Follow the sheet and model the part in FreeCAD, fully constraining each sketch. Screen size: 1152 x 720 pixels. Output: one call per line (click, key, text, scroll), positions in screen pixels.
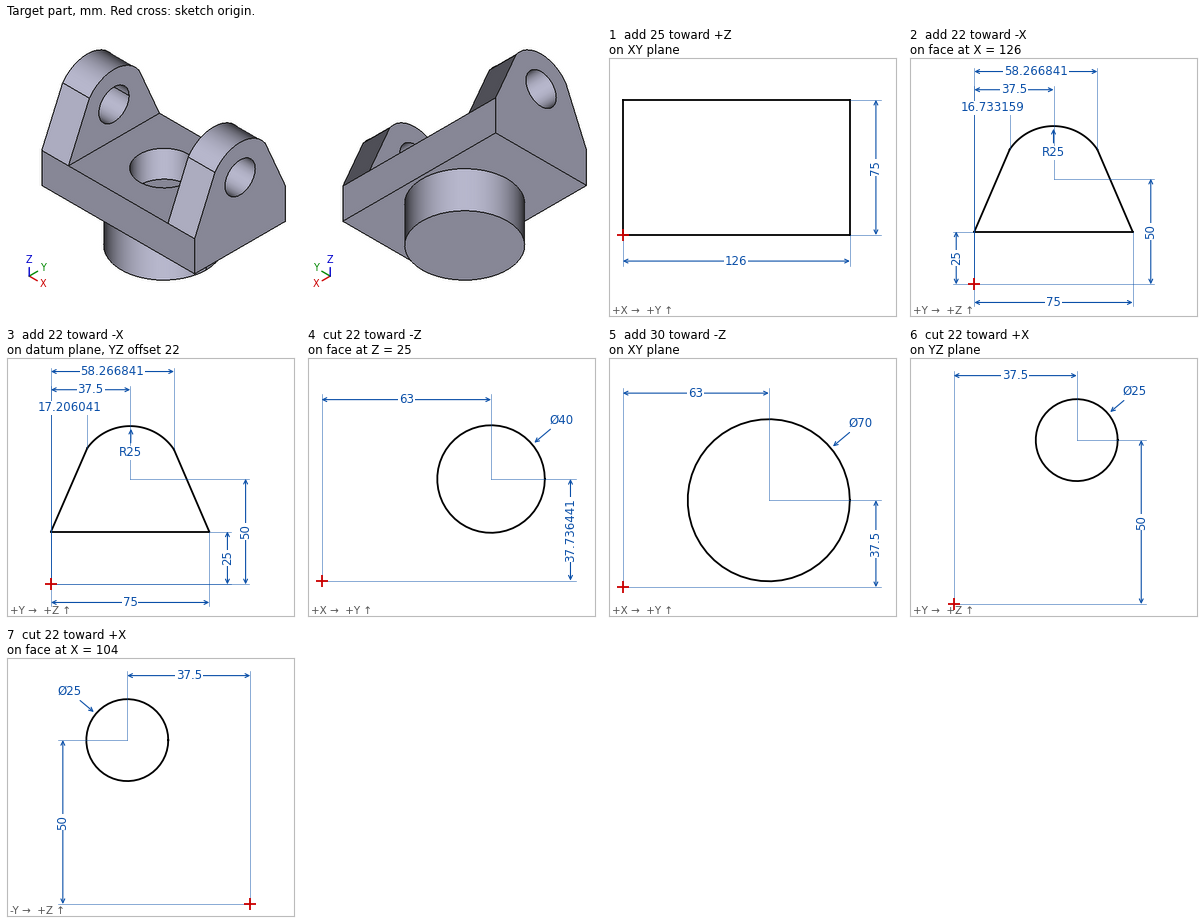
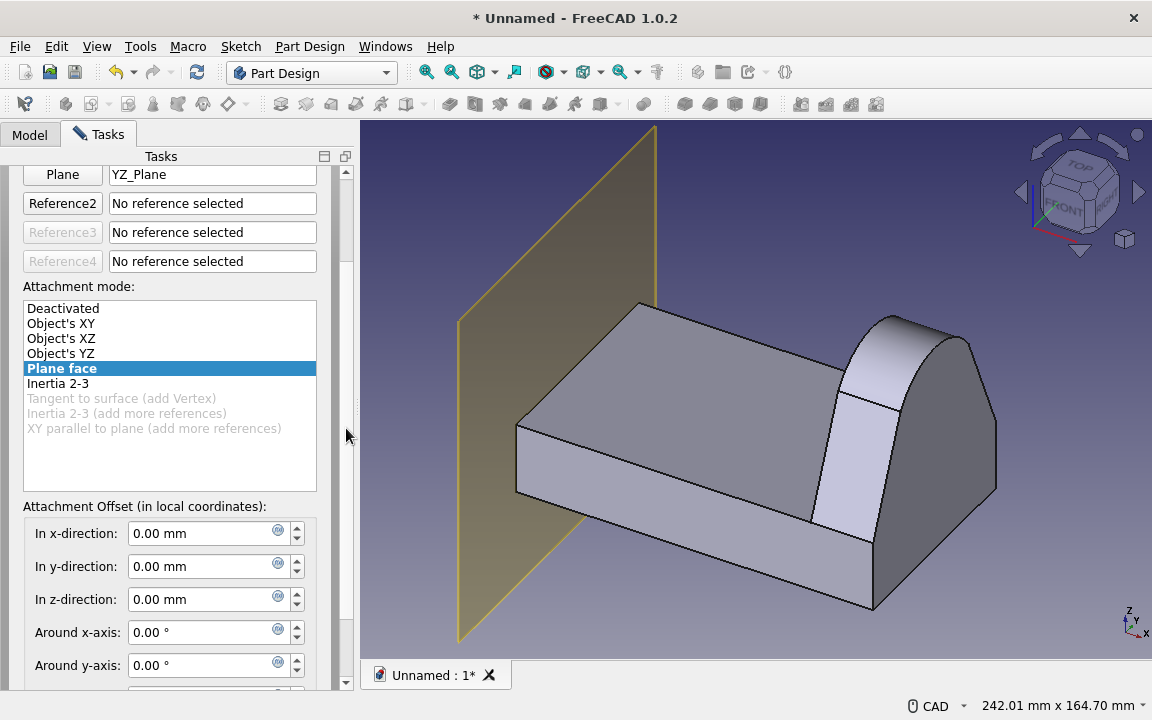
triple_click(210, 600)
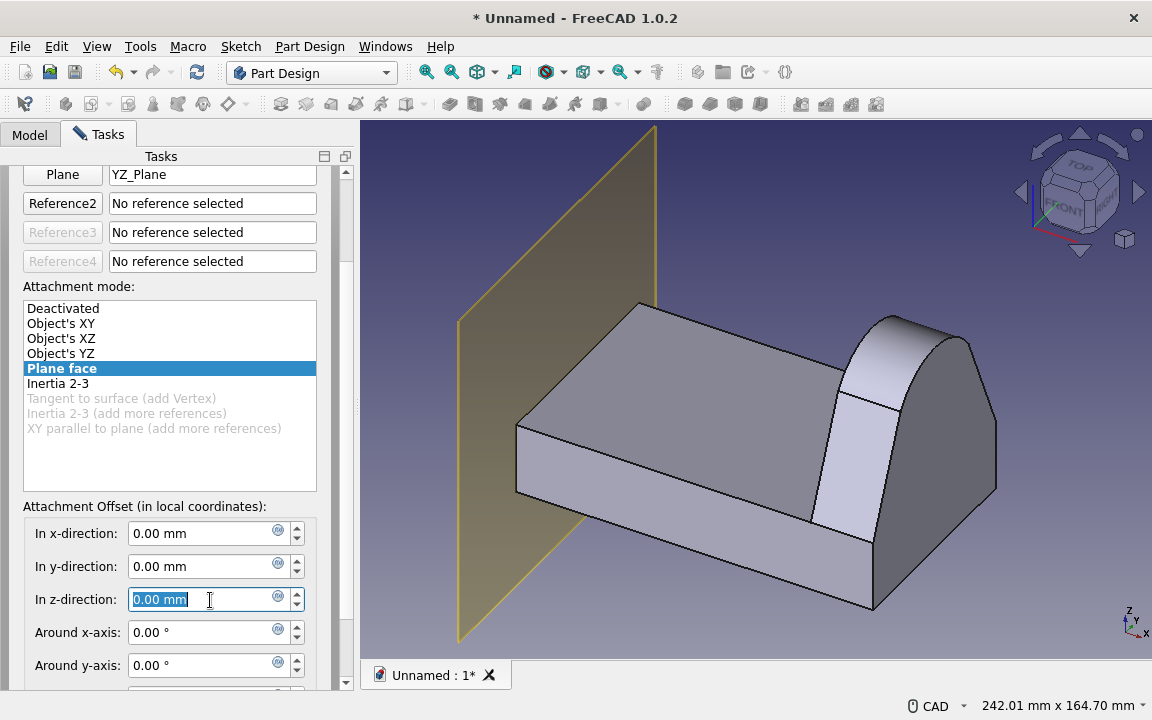
text(22)
key(Tab)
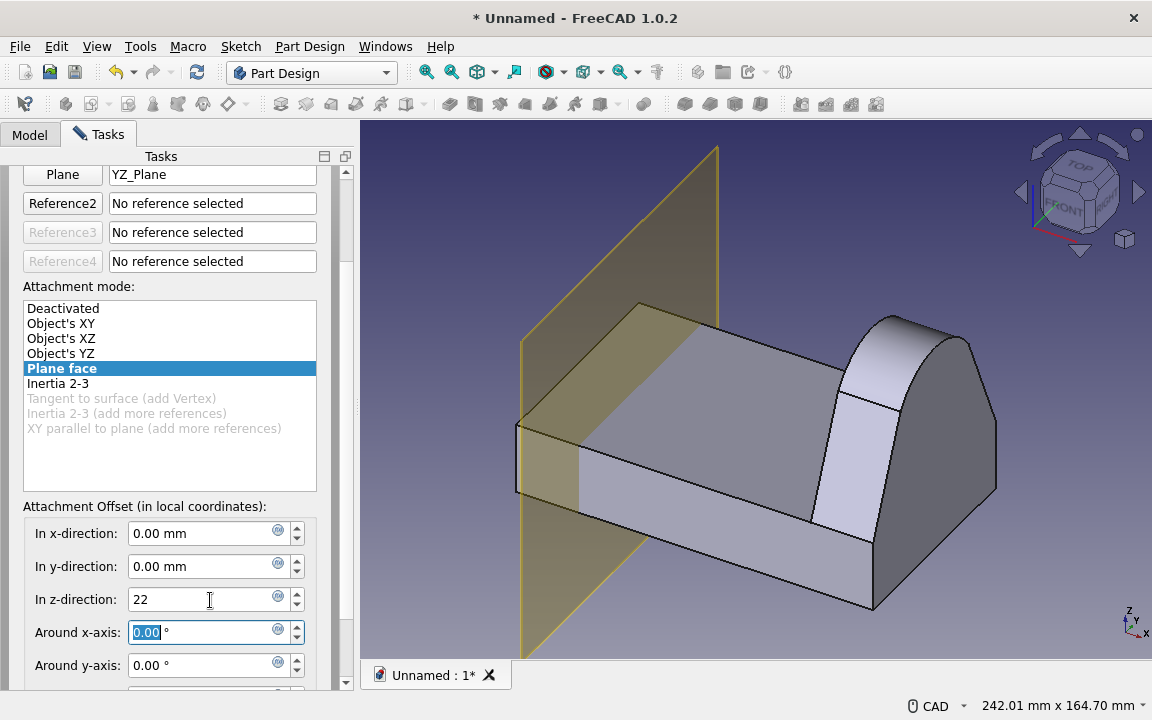
scroll(346, 428, up, 3)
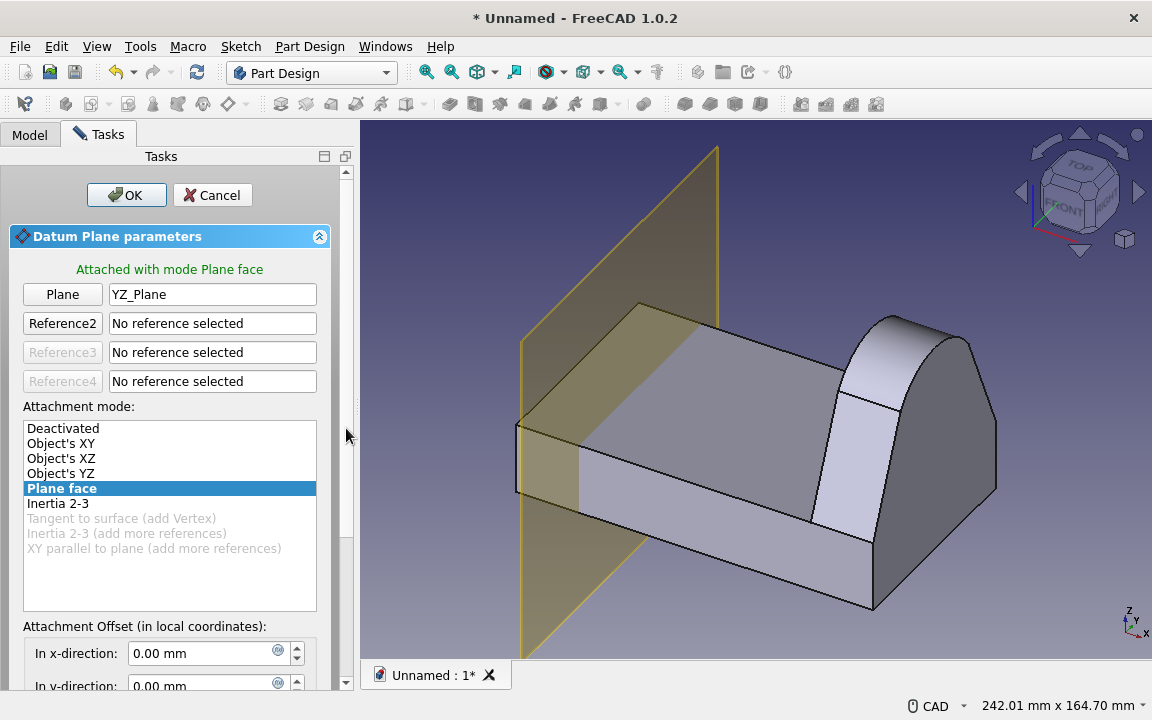
click(127, 195)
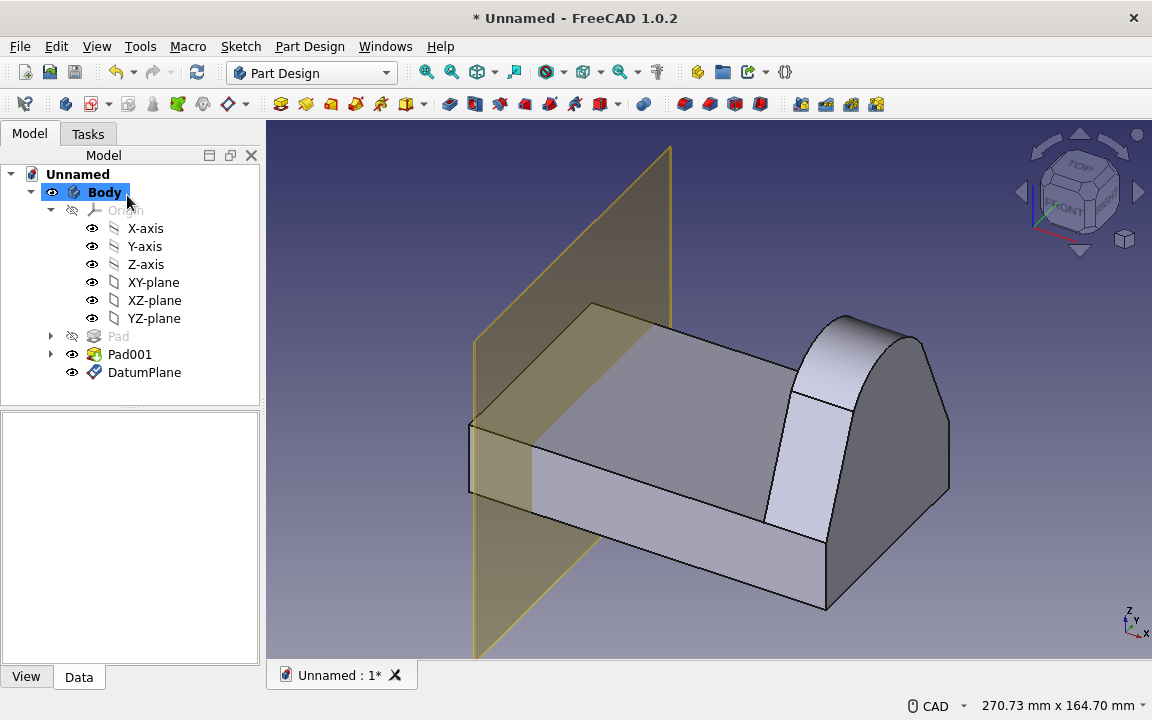
click(117, 372)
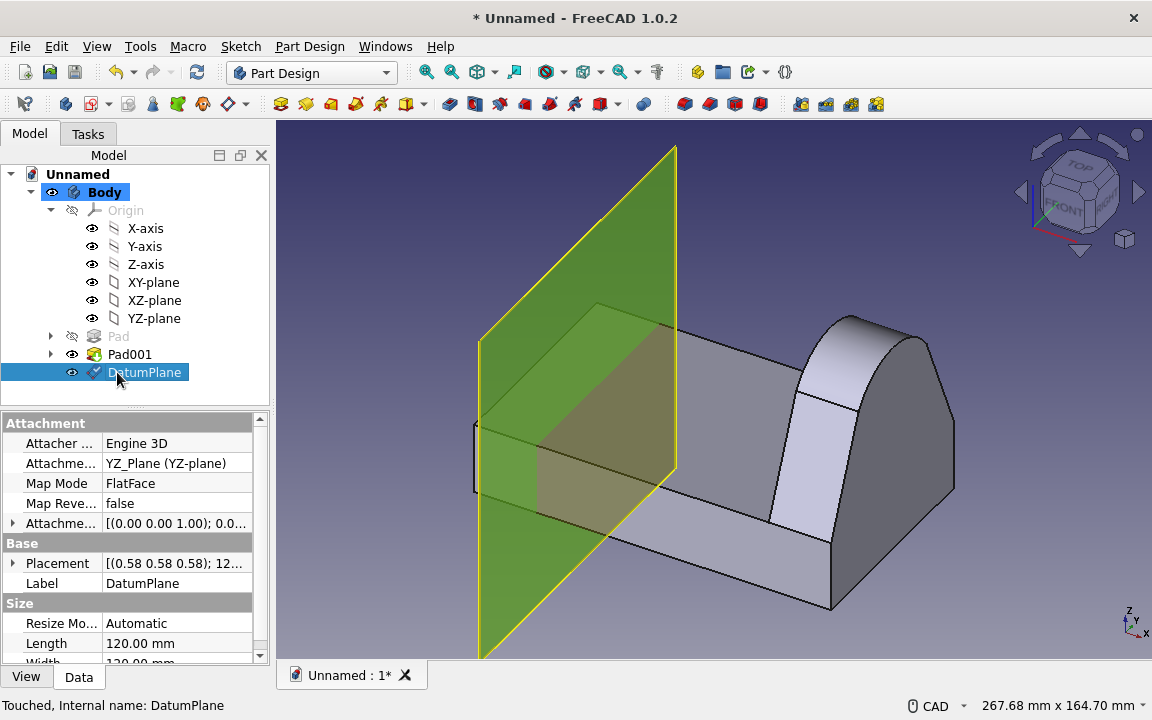
click(90, 104)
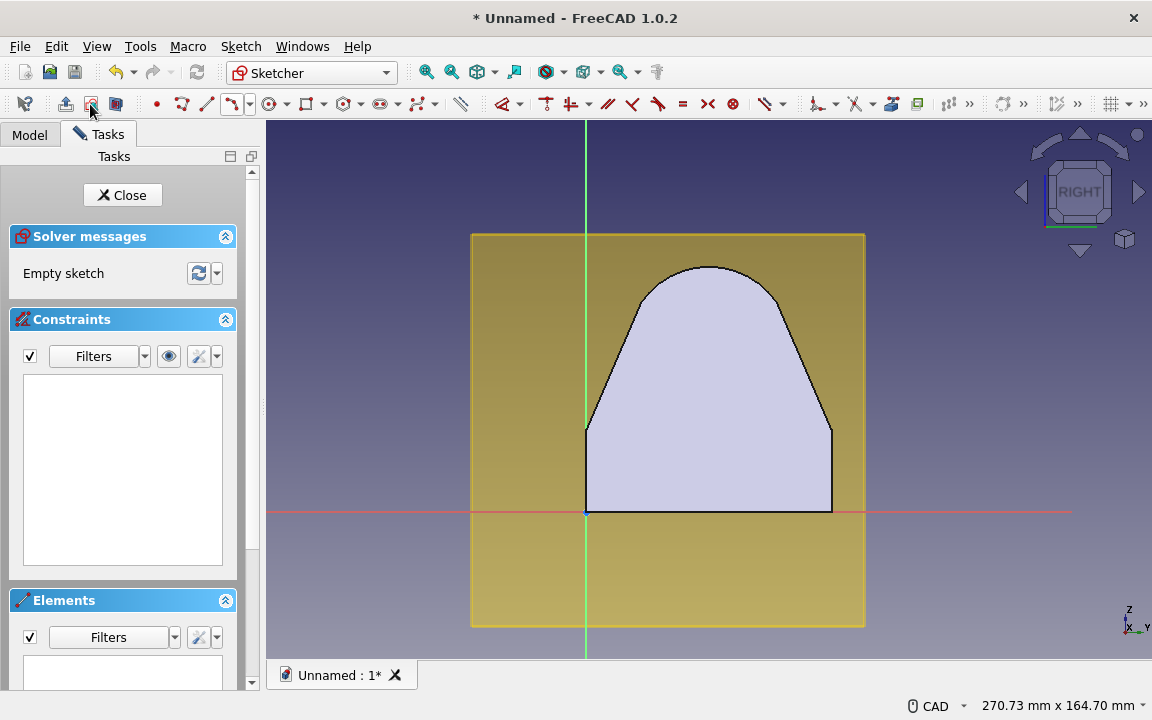
click(116, 104)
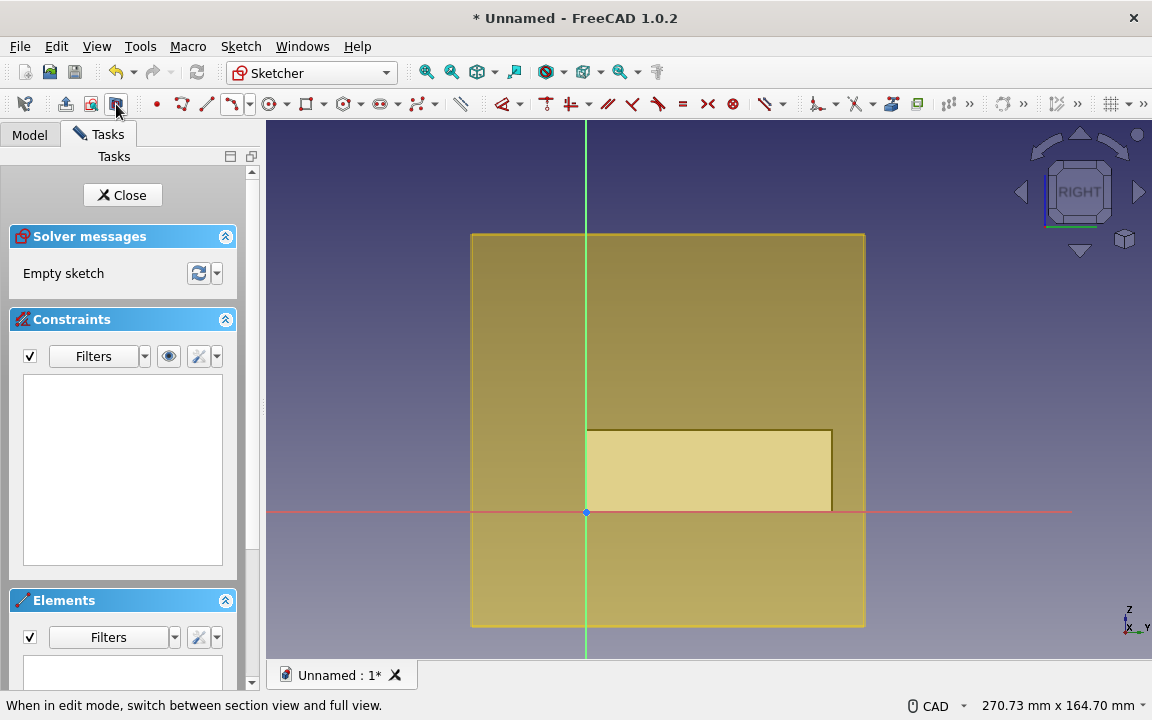
scroll(848, 390, up, 2)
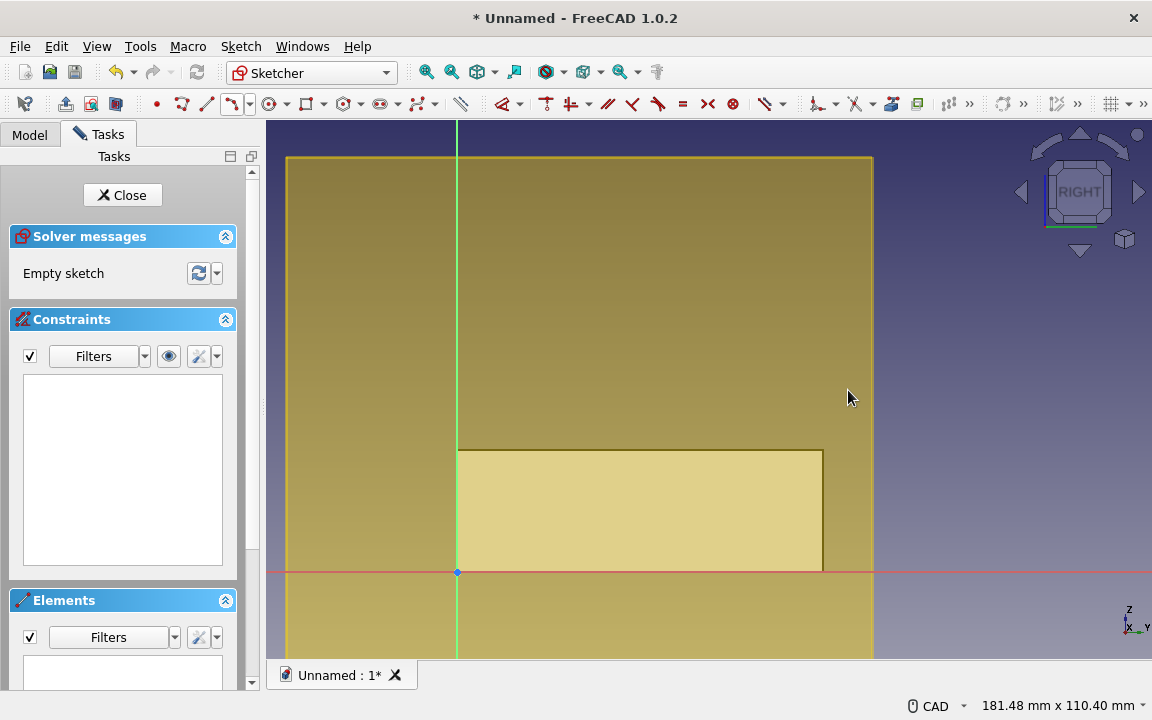
click(182, 104)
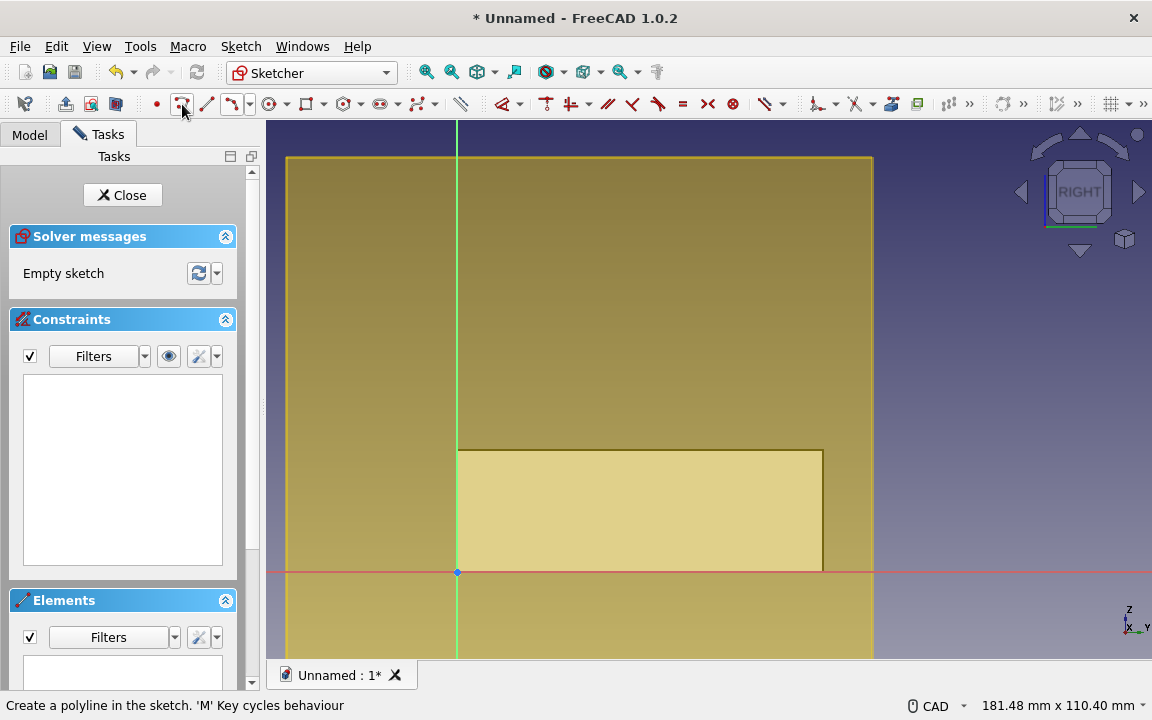
click(742, 260)
click(823, 450)
click(457, 450)
click(541, 257)
right_click(541, 257)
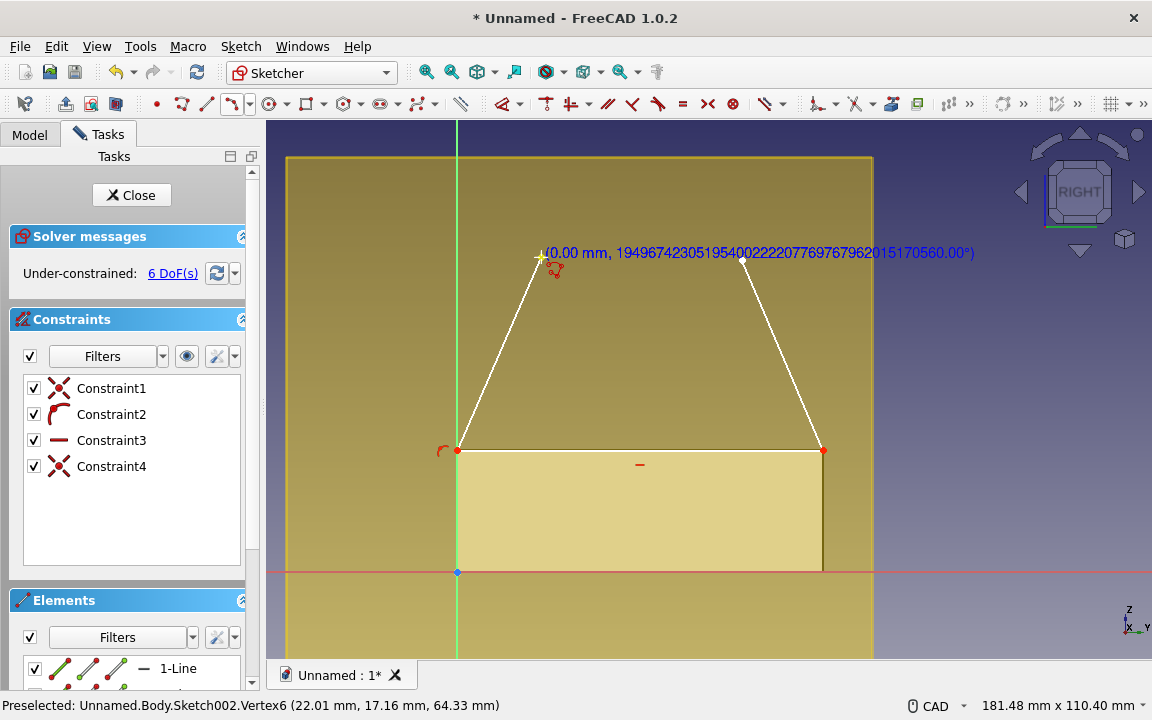
click(232, 104)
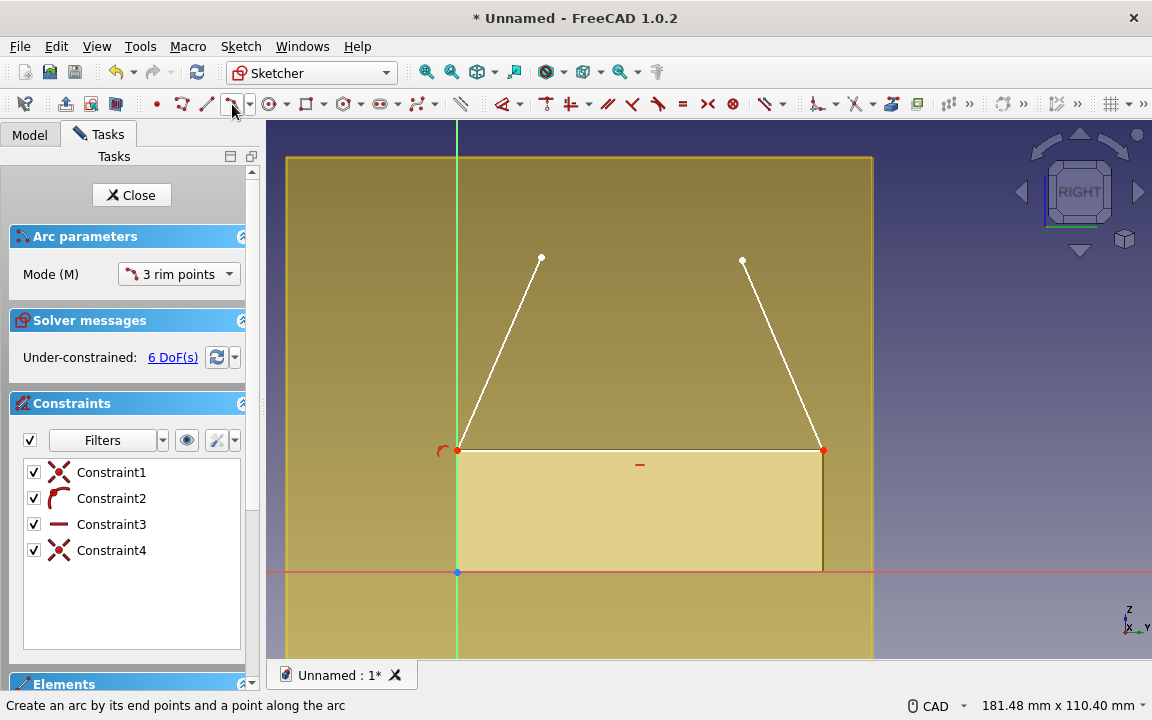
click(541, 258)
click(742, 261)
click(642, 206)
key(Escape)